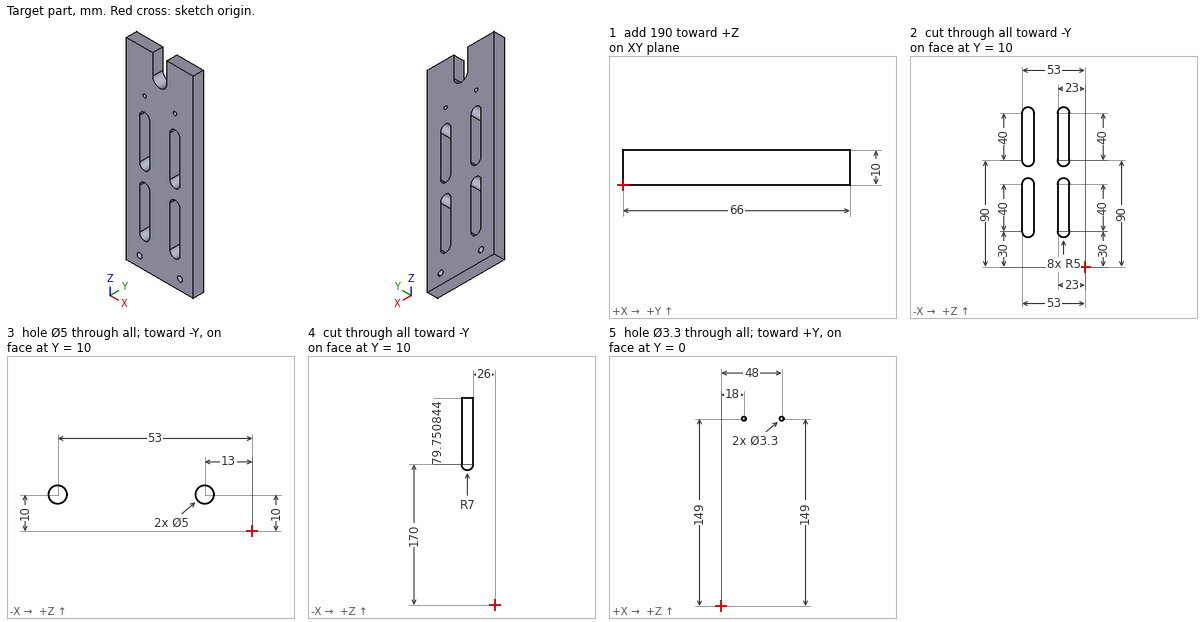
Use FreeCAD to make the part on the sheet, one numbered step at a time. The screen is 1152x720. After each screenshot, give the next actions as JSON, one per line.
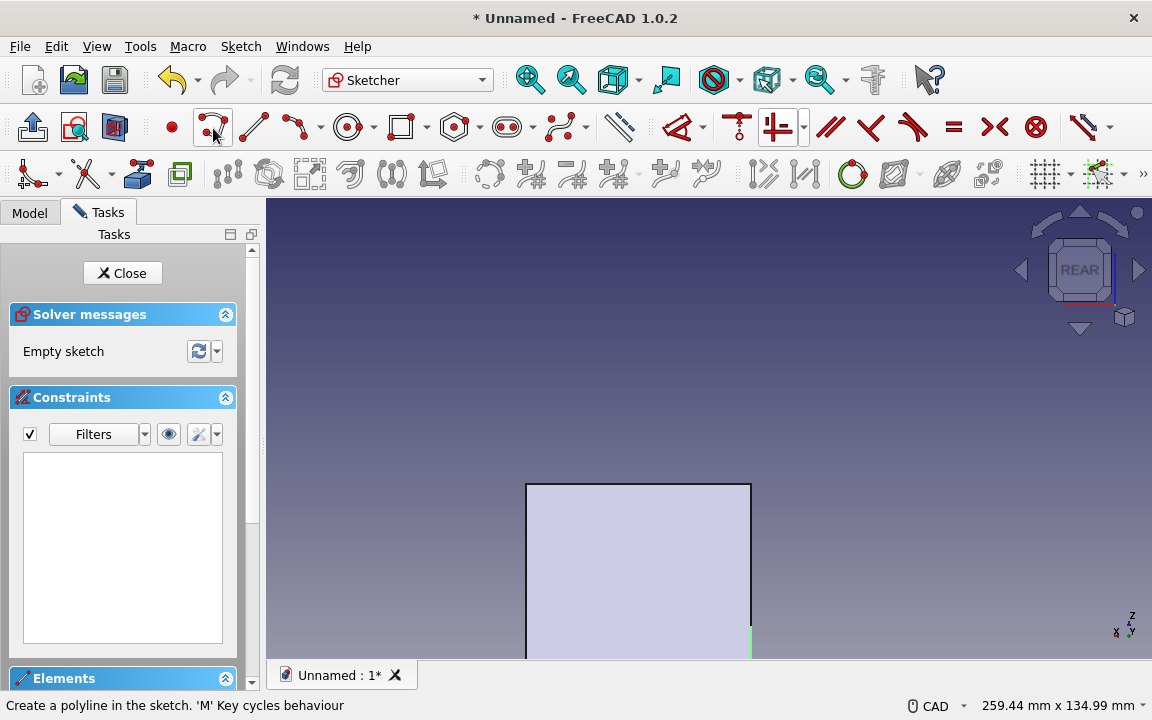
{"action": "left_click", "coordinate": [663, 552]}
{"action": "left_click", "coordinate": [663, 280]}
{"action": "left_click", "coordinate": [615, 280]}
{"action": "left_click", "coordinate": [615, 552]}
{"action": "right_click", "coordinate": [615, 552]}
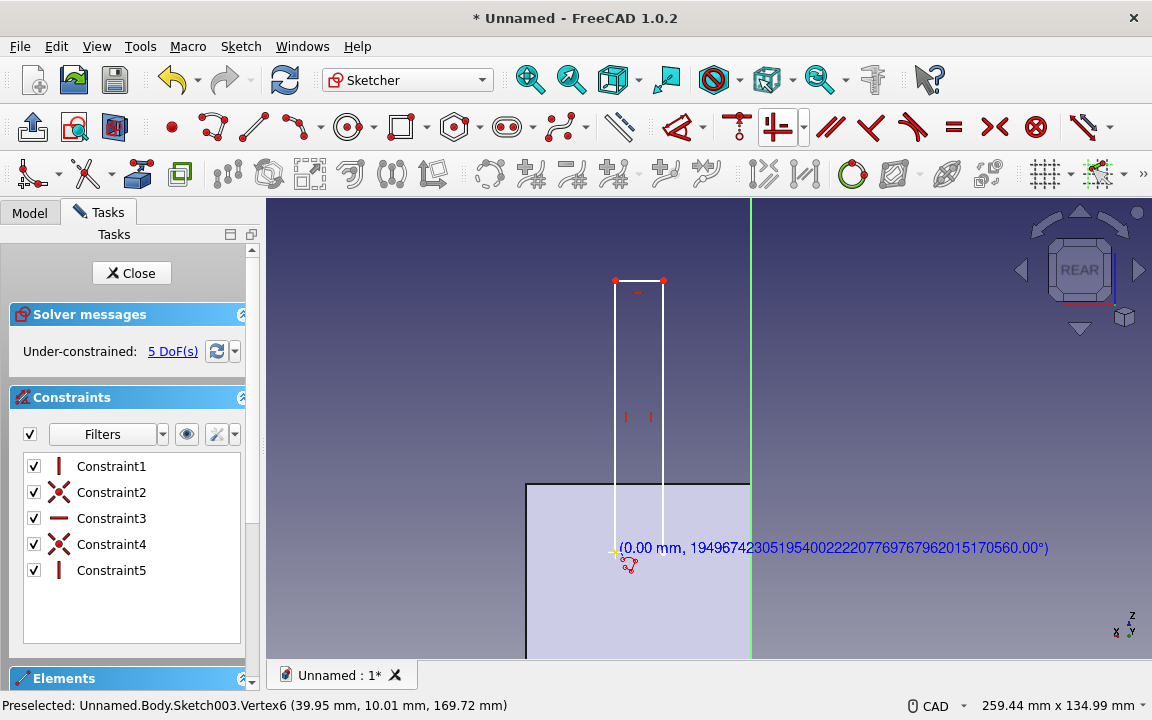
{"action": "left_click", "coordinate": [294, 128]}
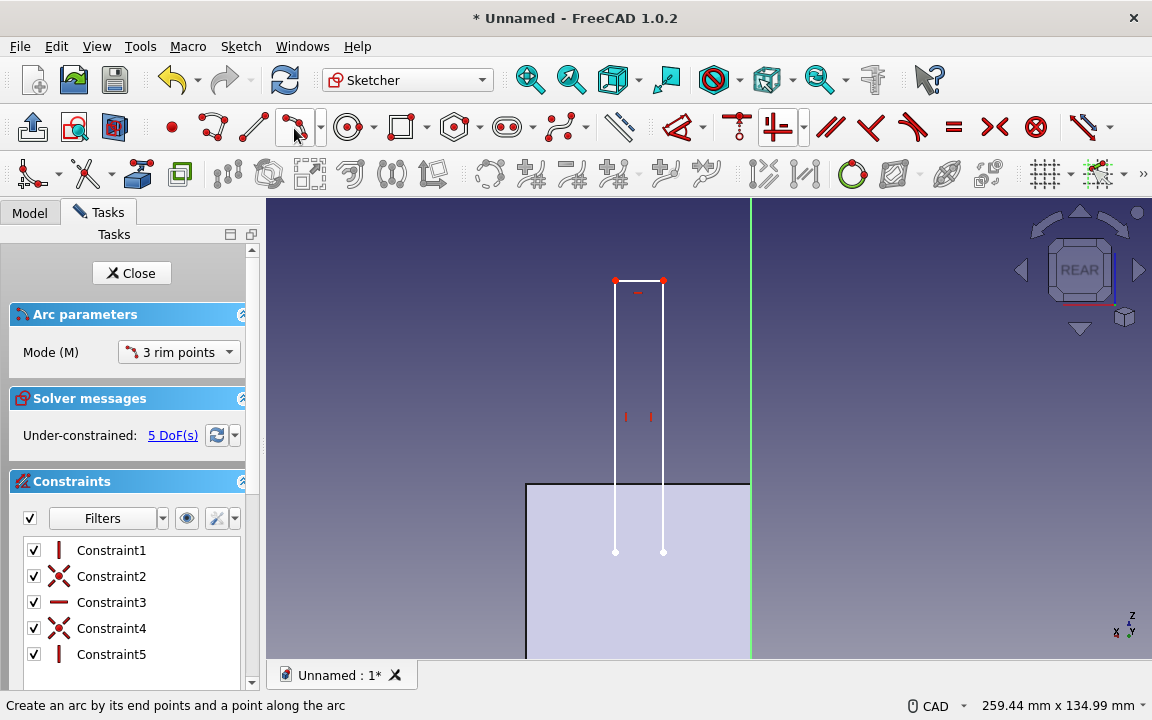
{"action": "left_click", "coordinate": [615, 553]}
{"action": "left_click", "coordinate": [663, 553]}
{"action": "left_click", "coordinate": [639, 576]}
{"action": "key", "text": "Escape"}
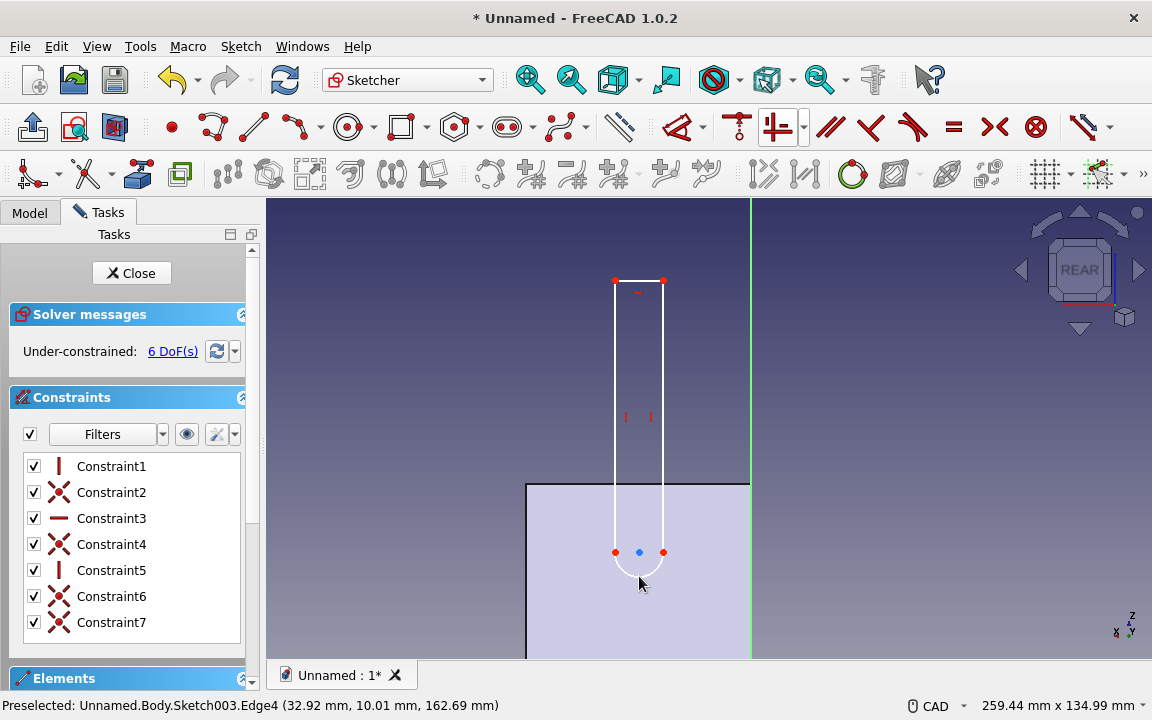
{"action": "left_click", "coordinate": [663, 471]}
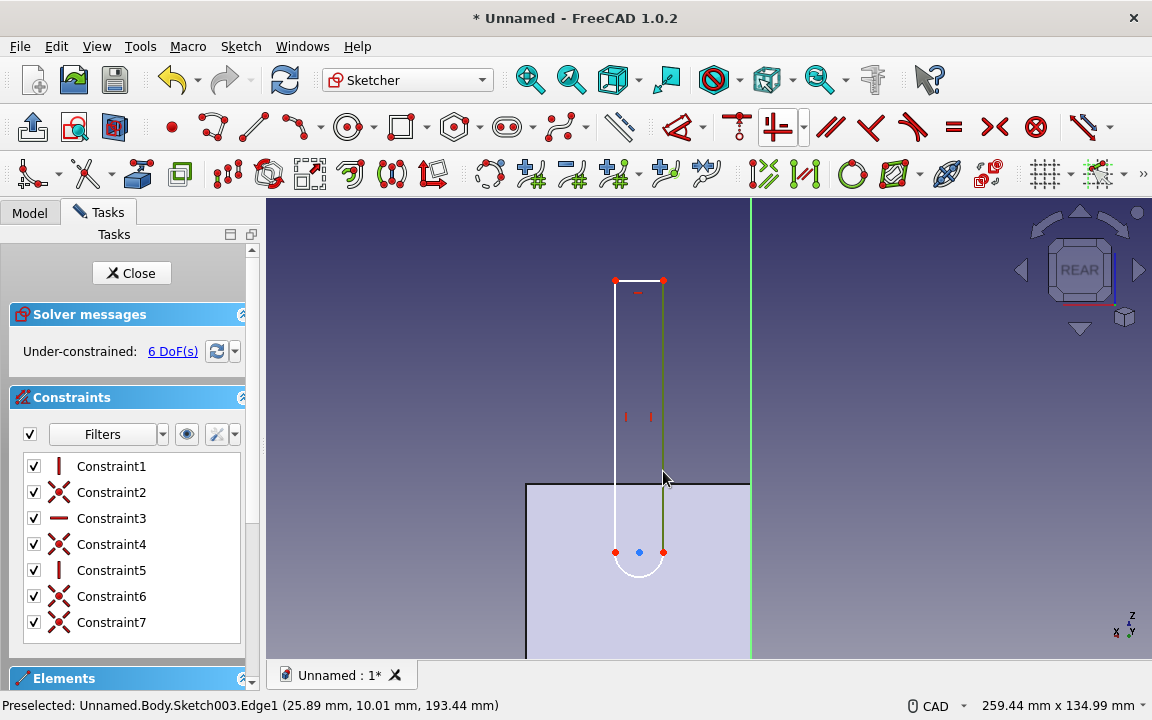
{"action": "left_click", "coordinate": [625, 572]}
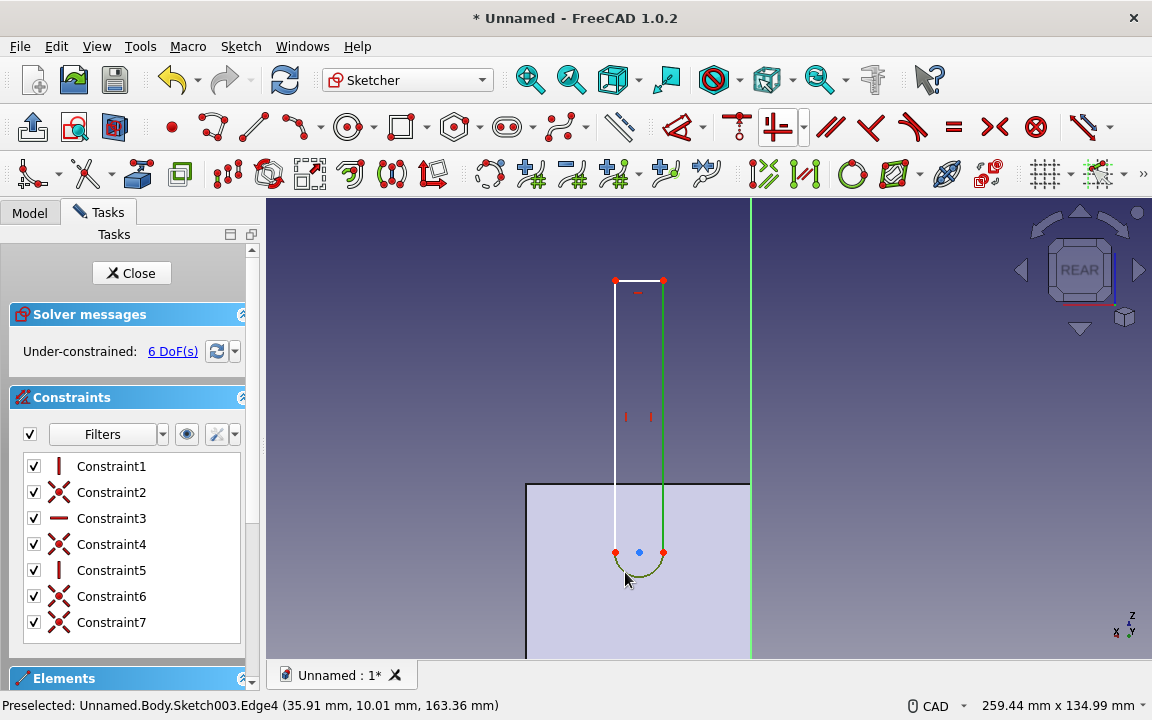
{"action": "left_click", "coordinate": [913, 128]}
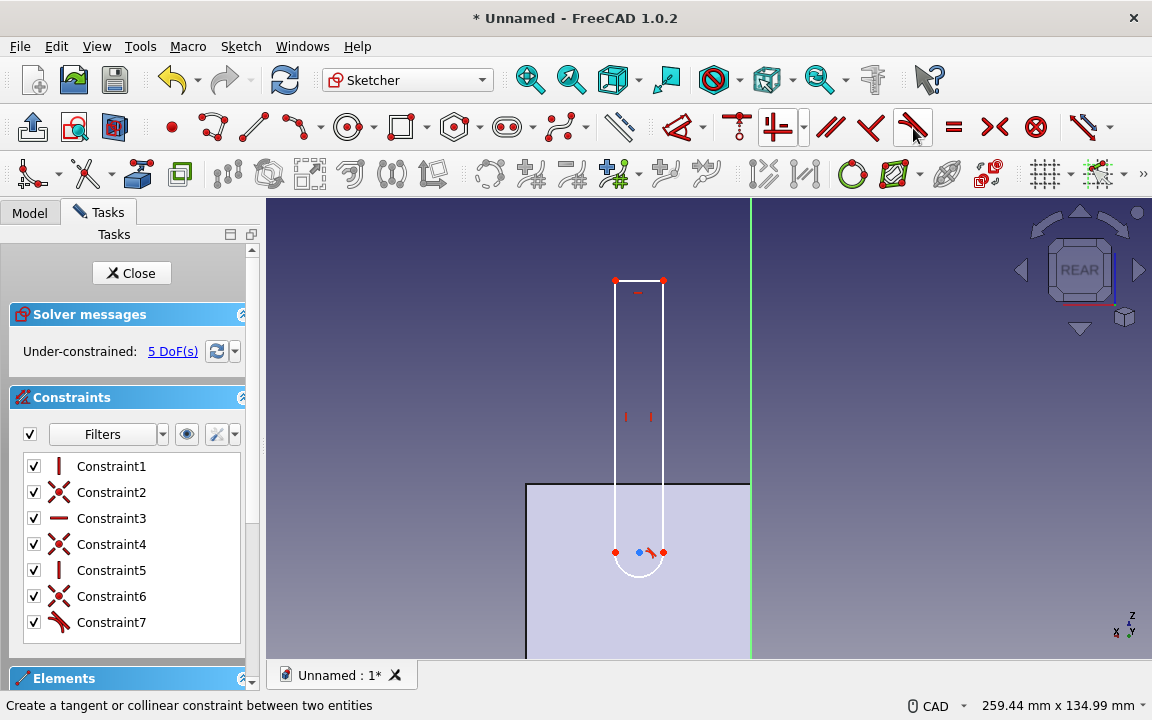
{"action": "left_click", "coordinate": [615, 363]}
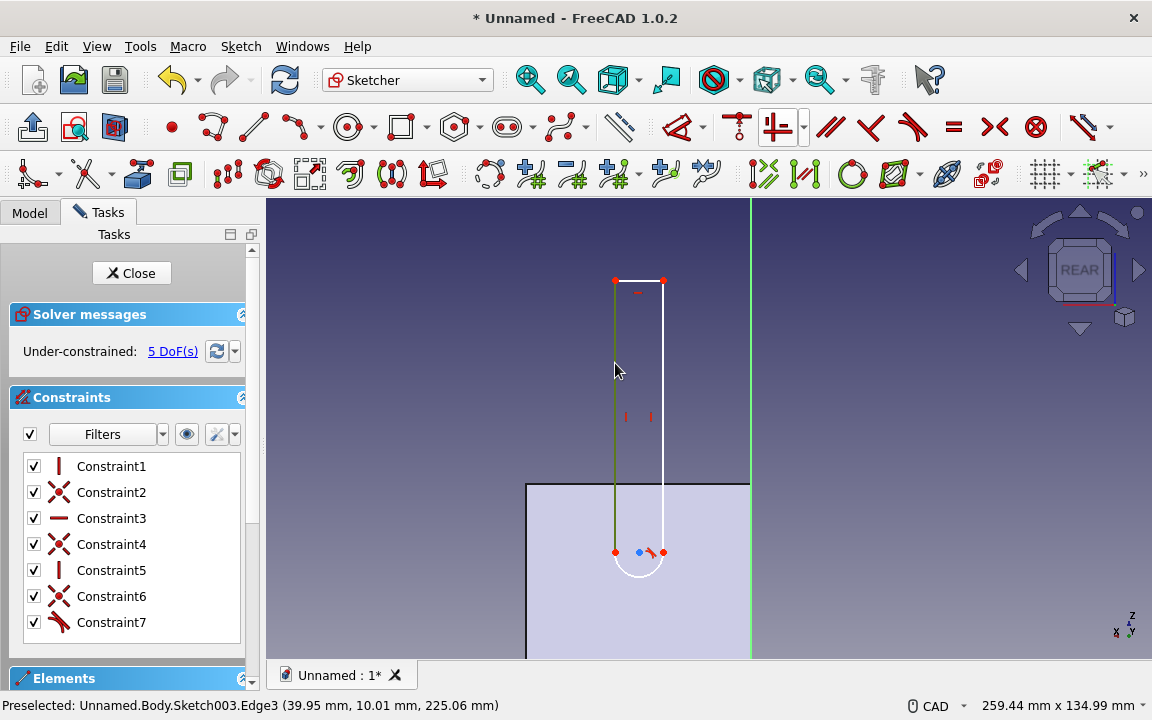
{"action": "left_click", "coordinate": [625, 572]}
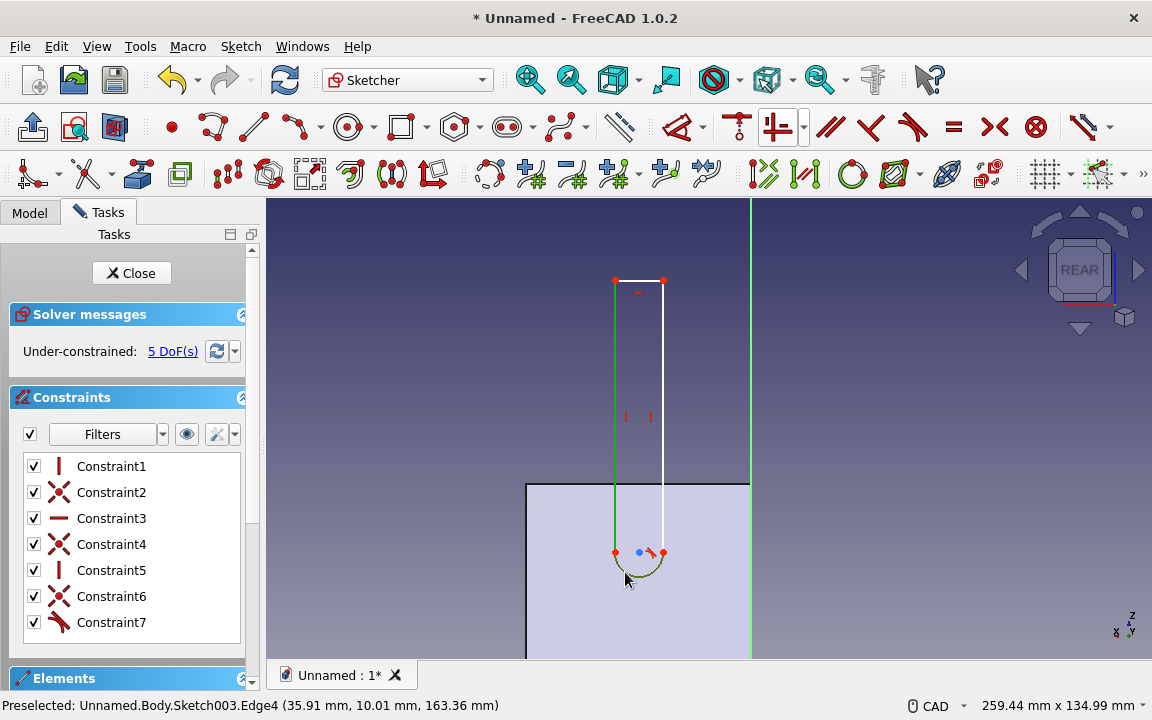
{"action": "left_click", "coordinate": [913, 128]}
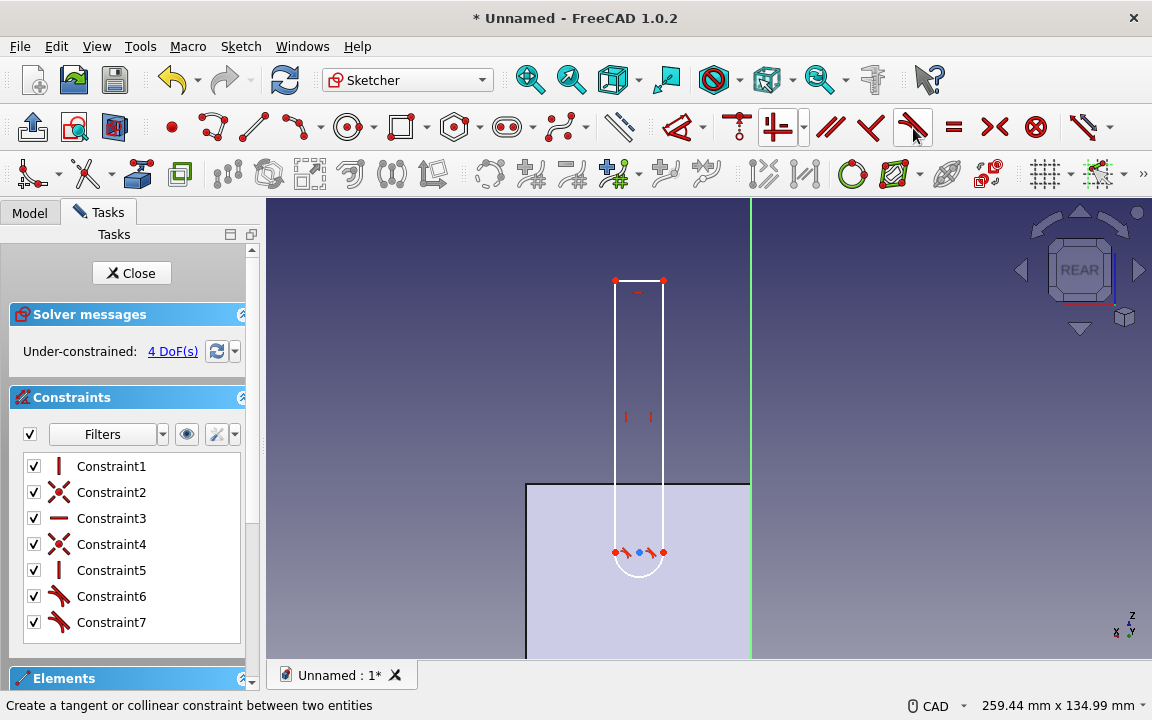
{"action": "left_click", "coordinate": [676, 128]}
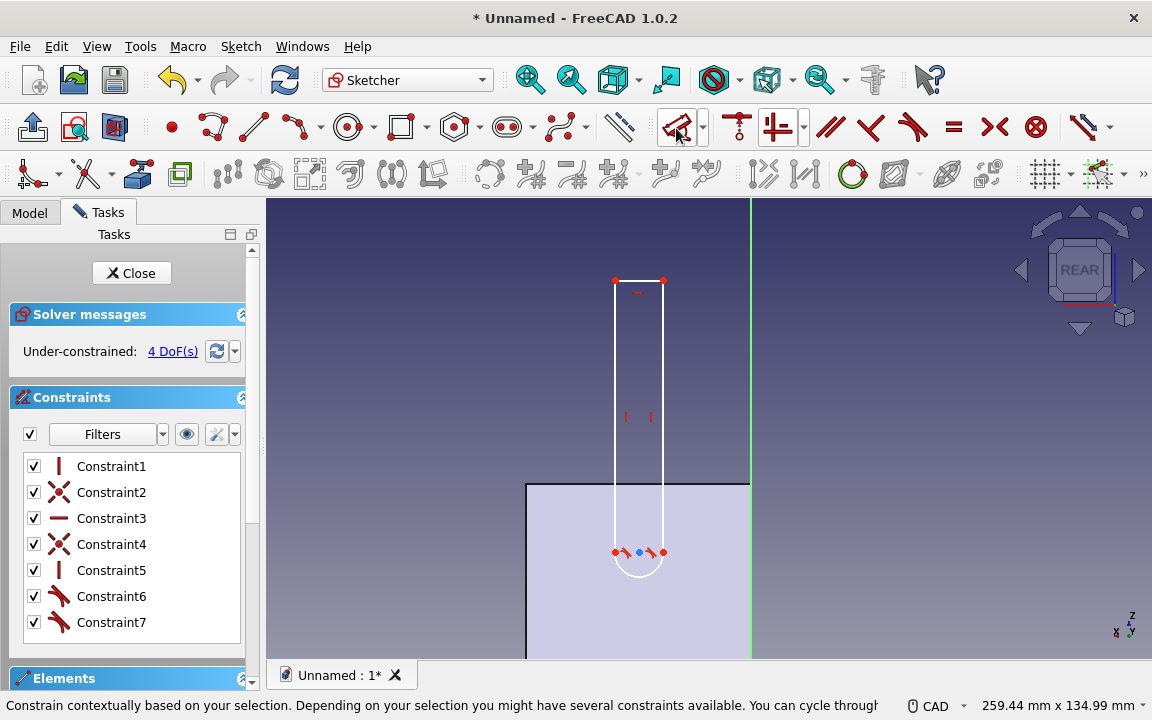
{"action": "scroll", "coordinate": [625, 572], "scroll_direction": "up", "scroll_amount": 3}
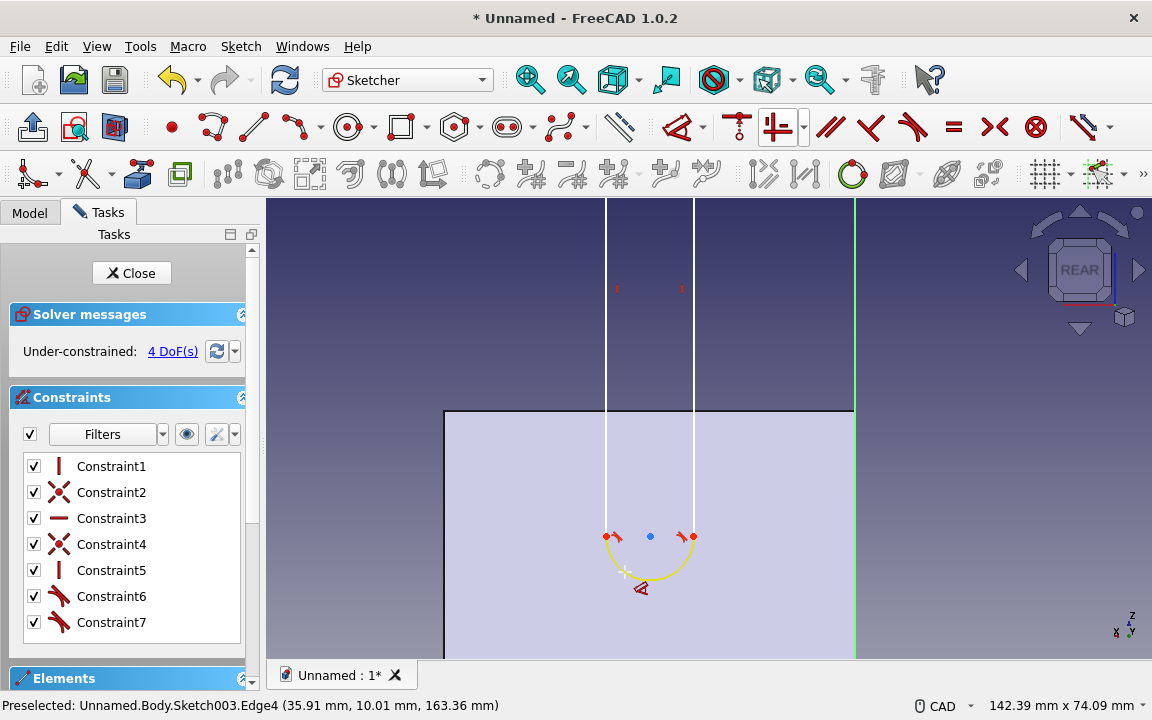
{"action": "left_click", "coordinate": [624, 572]}
{"action": "left_click", "coordinate": [605, 598]}